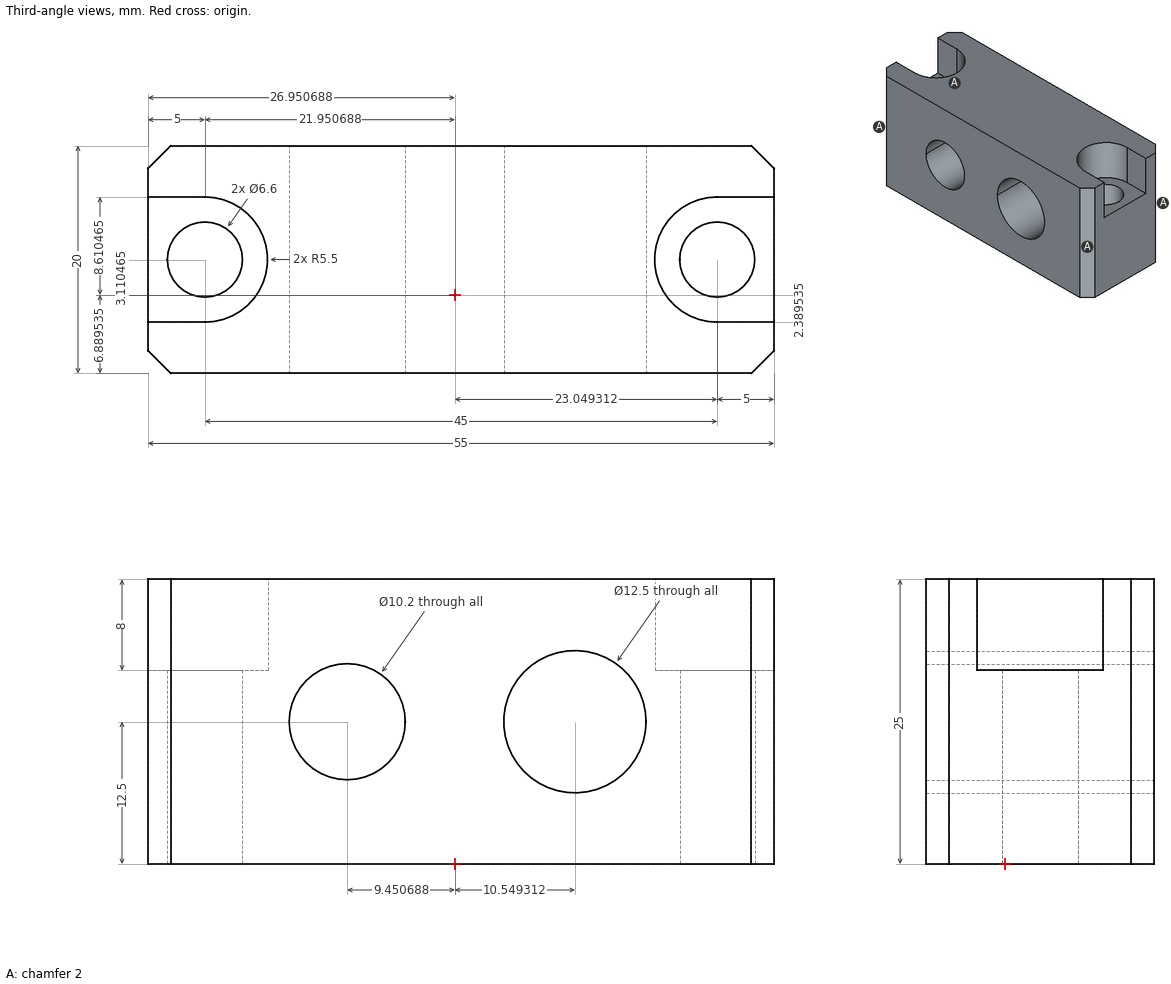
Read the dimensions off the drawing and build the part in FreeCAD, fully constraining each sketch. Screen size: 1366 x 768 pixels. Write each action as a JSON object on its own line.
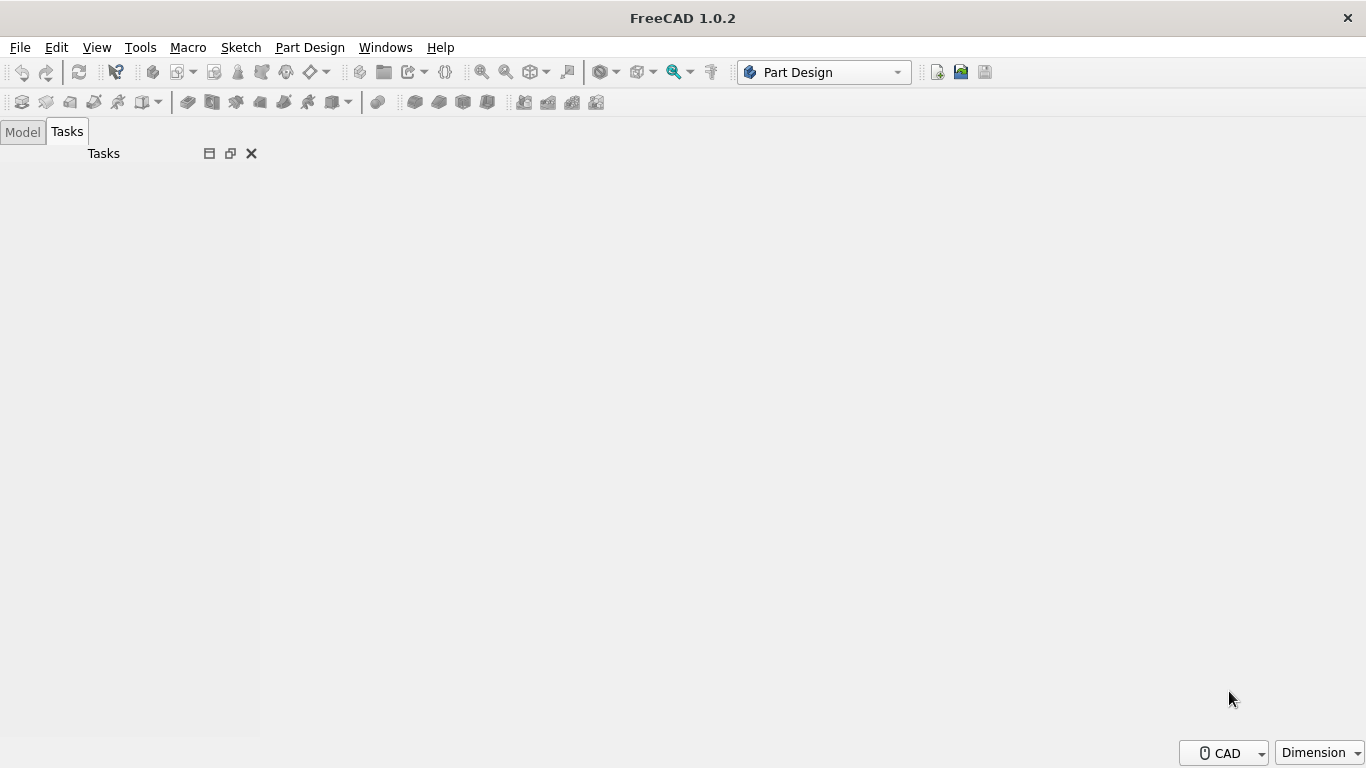
{"action": "left_click", "coordinate": [938, 72]}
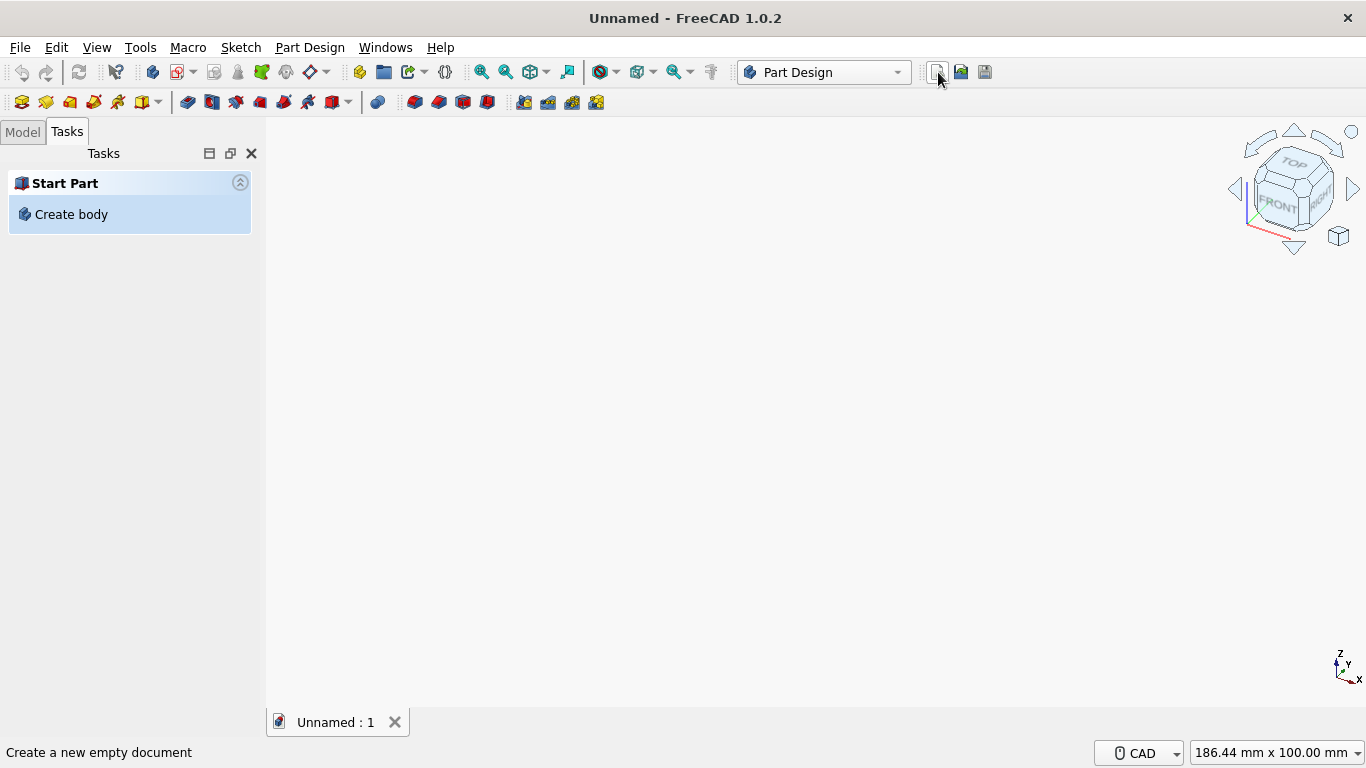
{"action": "left_click", "coordinate": [178, 72]}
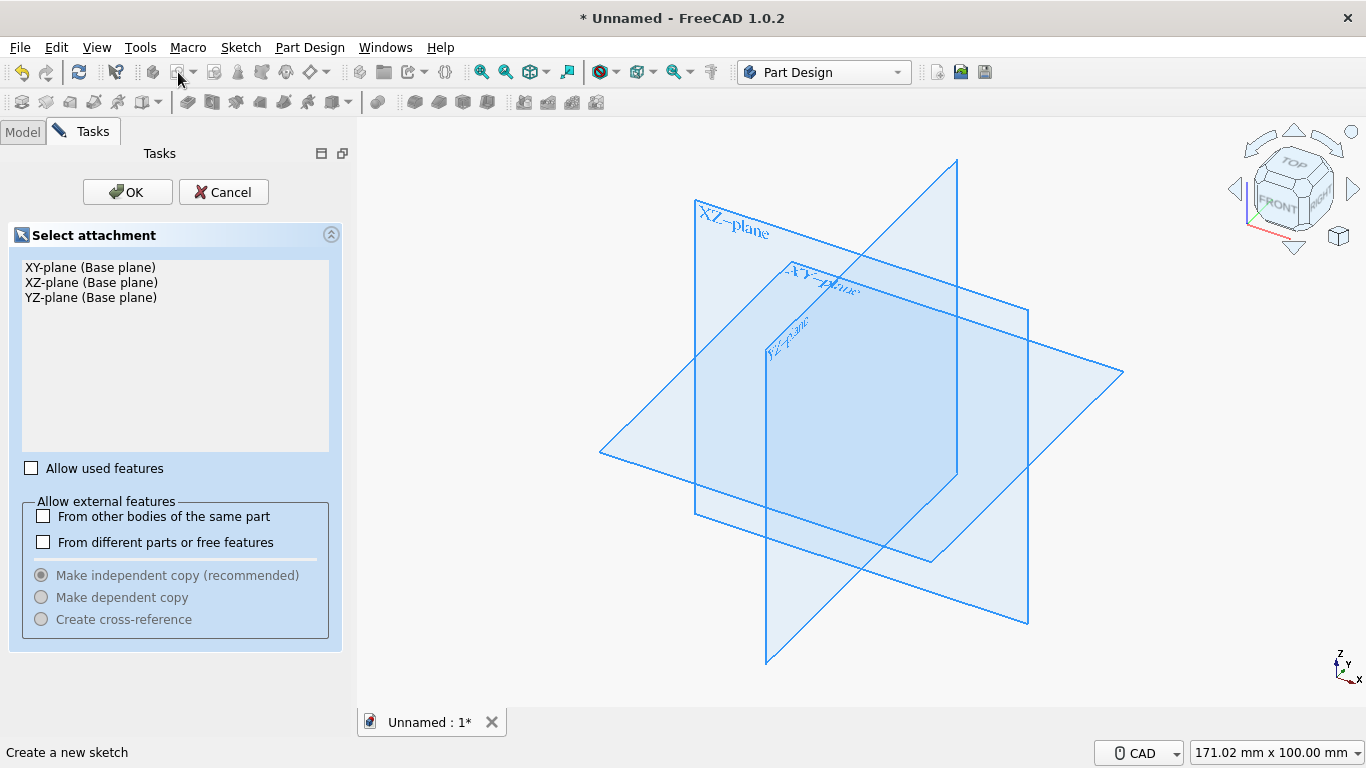
{"action": "left_click", "coordinate": [82, 268]}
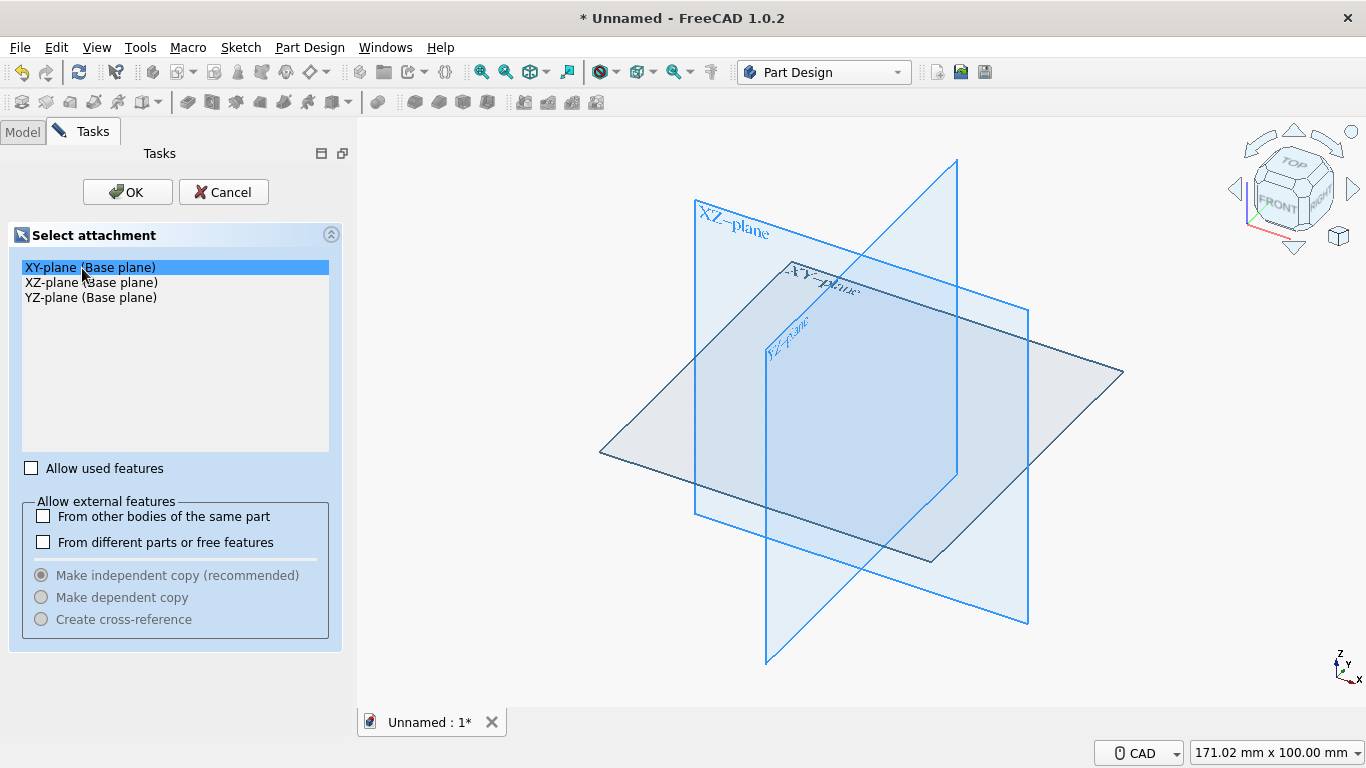
{"action": "left_click", "coordinate": [128, 192]}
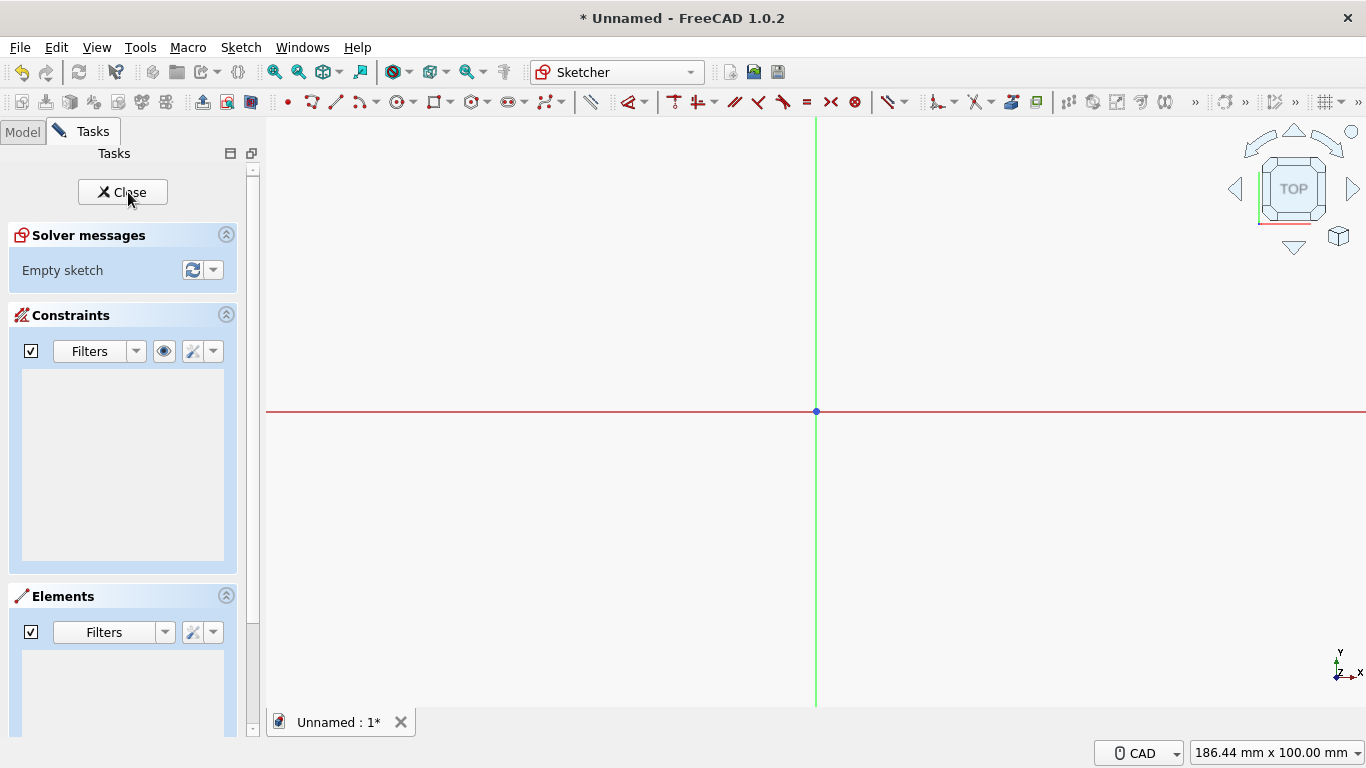
{"action": "scroll", "coordinate": [907, 371], "scroll_direction": "up", "scroll_amount": 3}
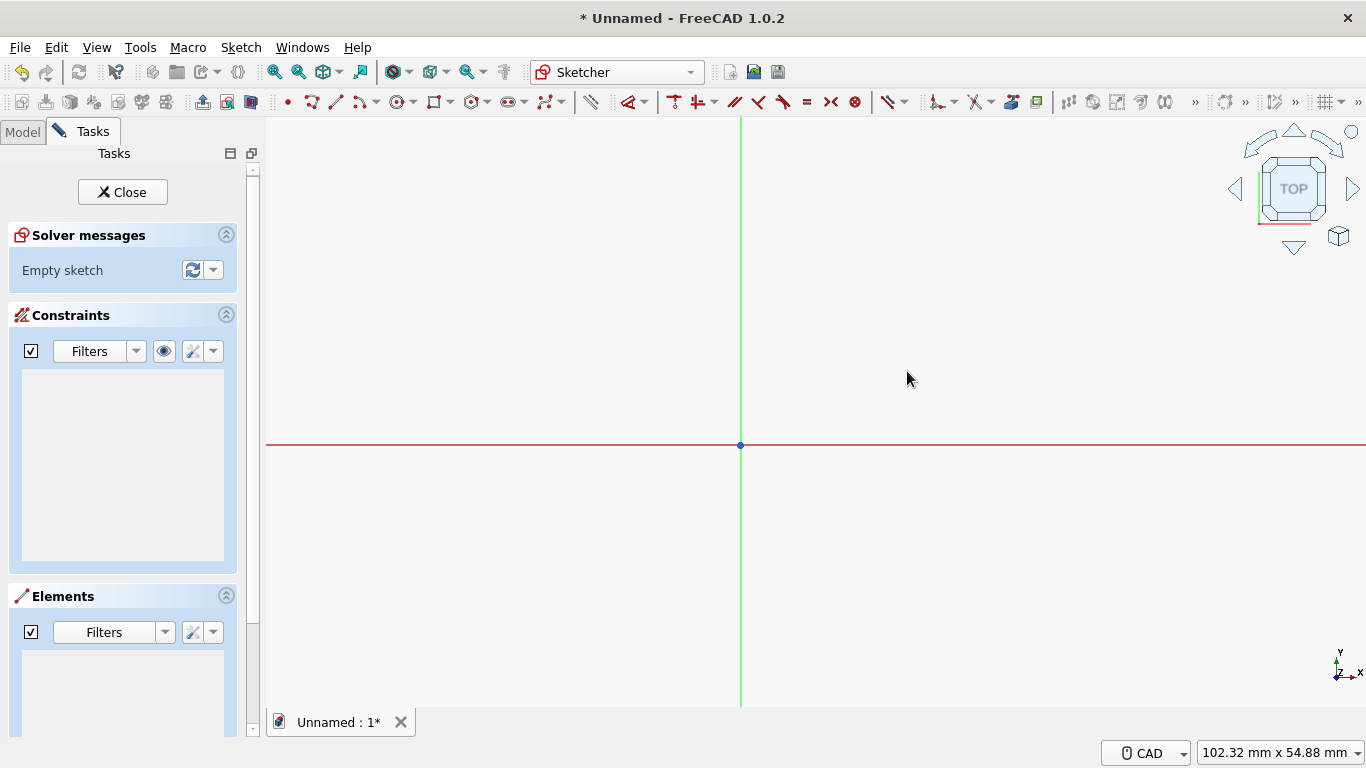
{"action": "left_click", "coordinate": [434, 102]}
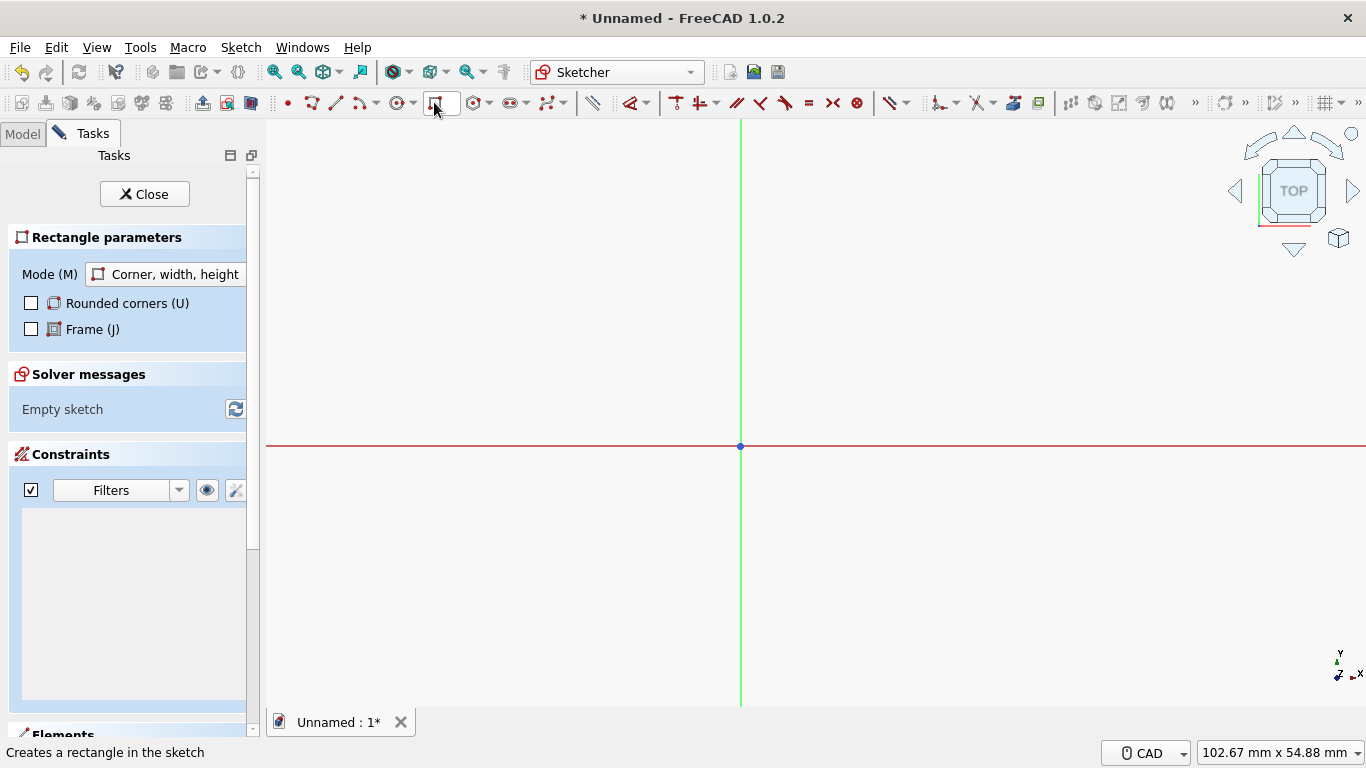
{"action": "left_click", "coordinate": [452, 306]}
{"action": "left_click", "coordinate": [1041, 520]}
{"action": "key", "text": "Escape"}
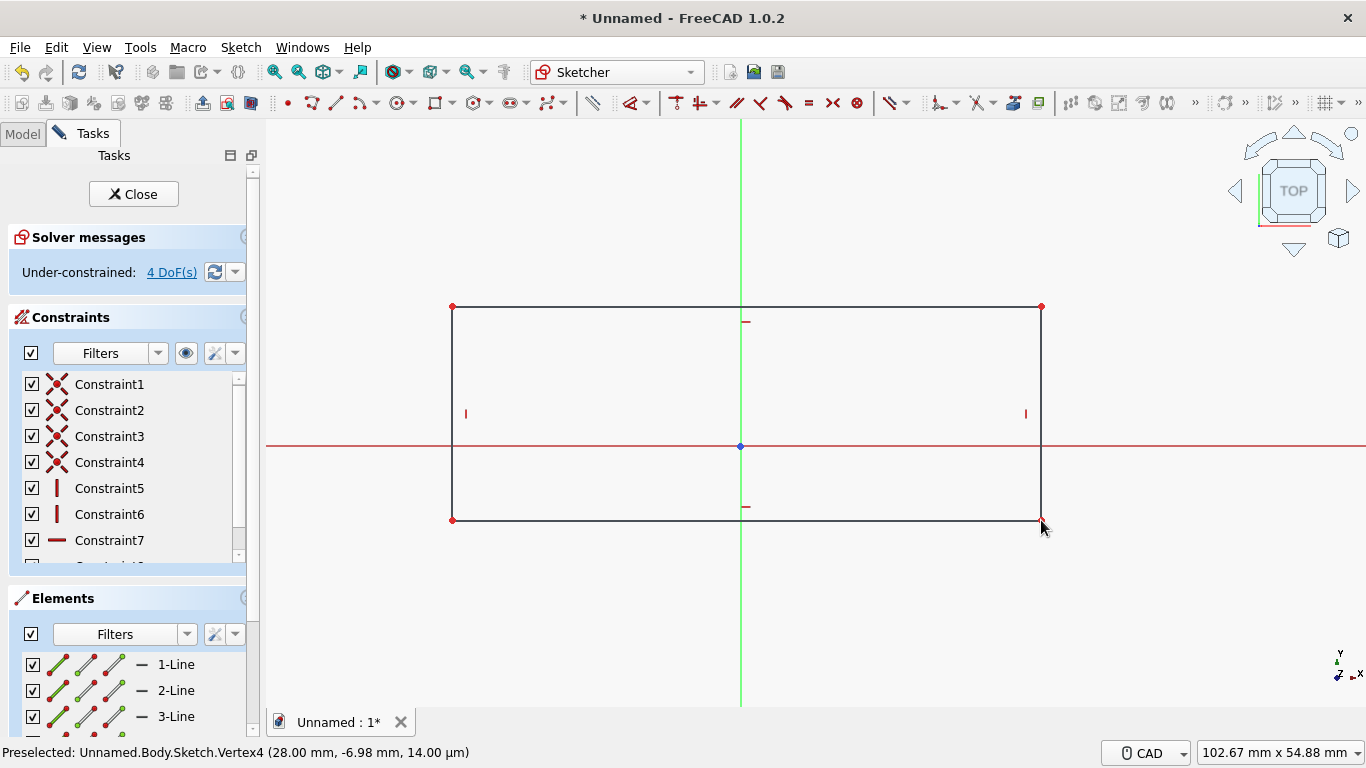
{"action": "key", "text": "d"}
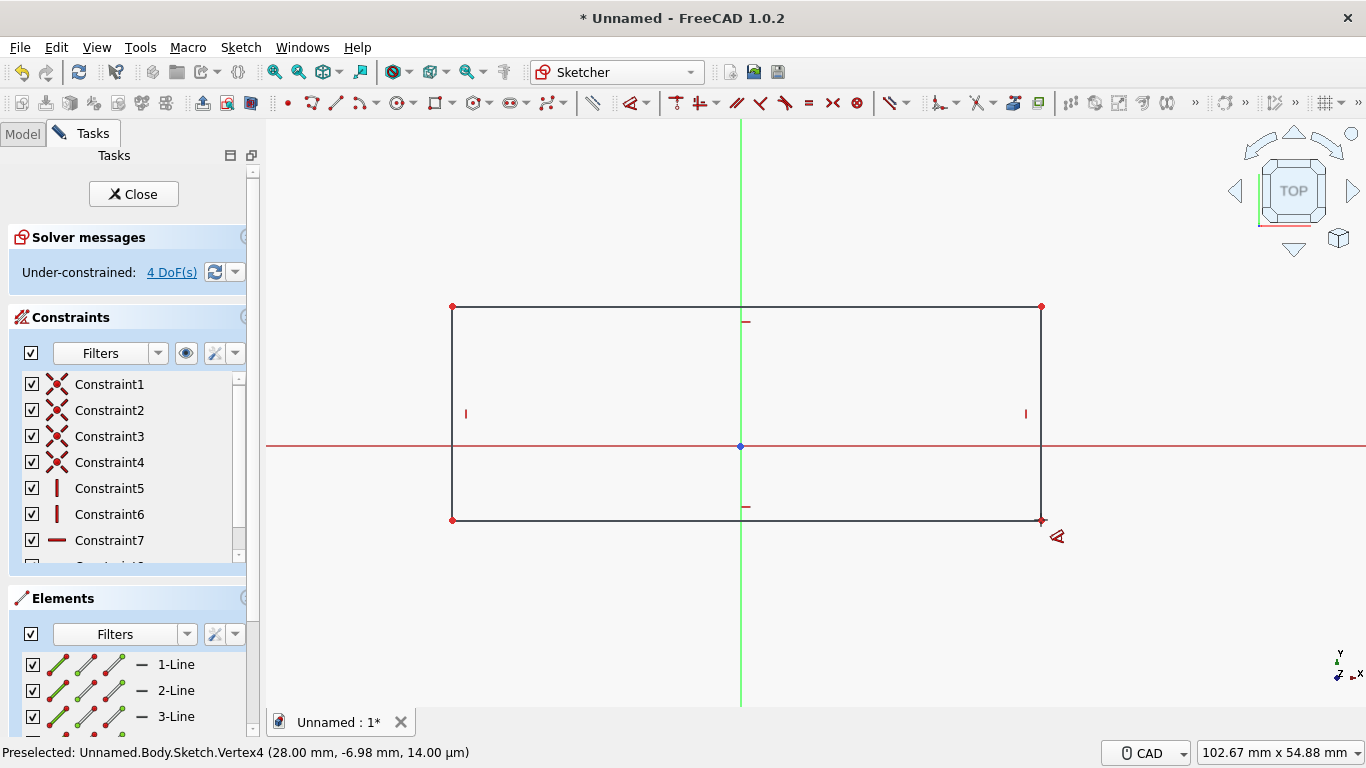
{"action": "left_click", "coordinate": [452, 371]}
{"action": "left_click", "coordinate": [418, 414]}